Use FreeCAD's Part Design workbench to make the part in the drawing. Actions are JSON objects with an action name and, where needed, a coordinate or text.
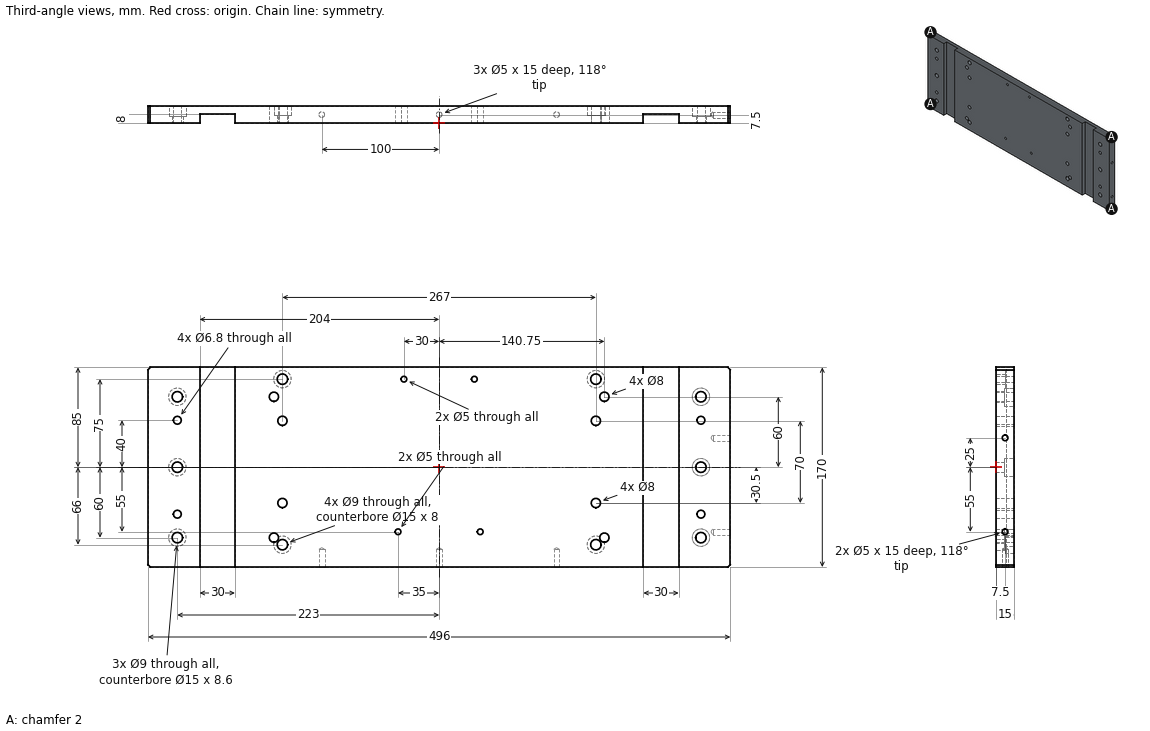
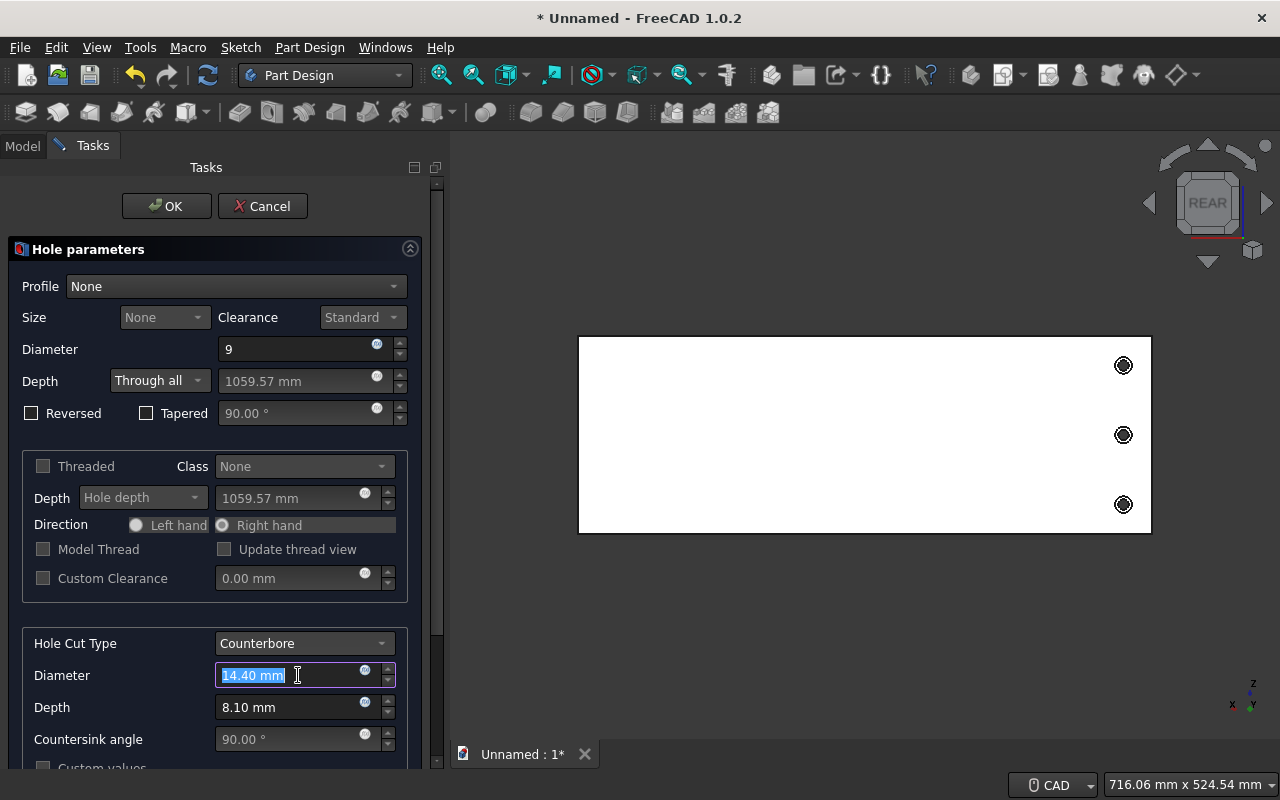
{"action": "type", "text": "15"}
{"action": "key", "text": "Tab"}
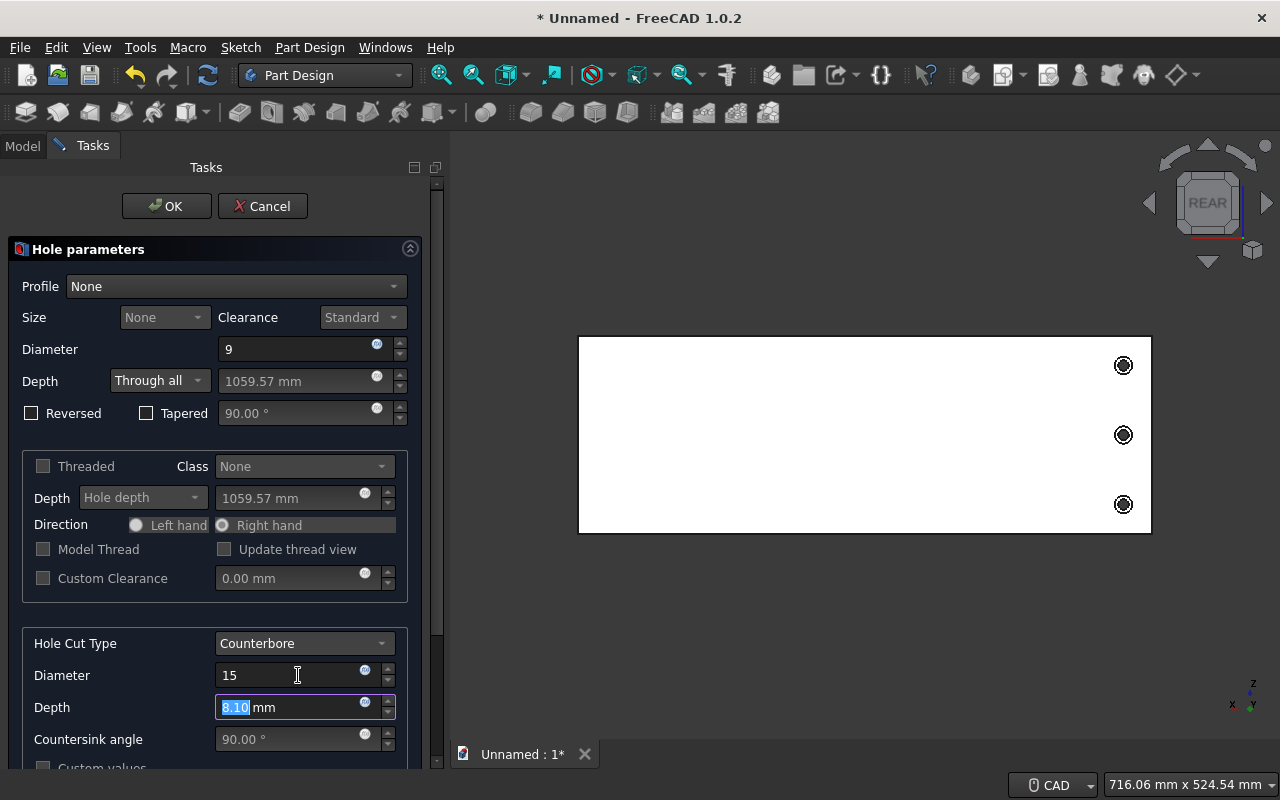
{"action": "type", "text": "8.6"}
{"action": "key", "text": "Tab"}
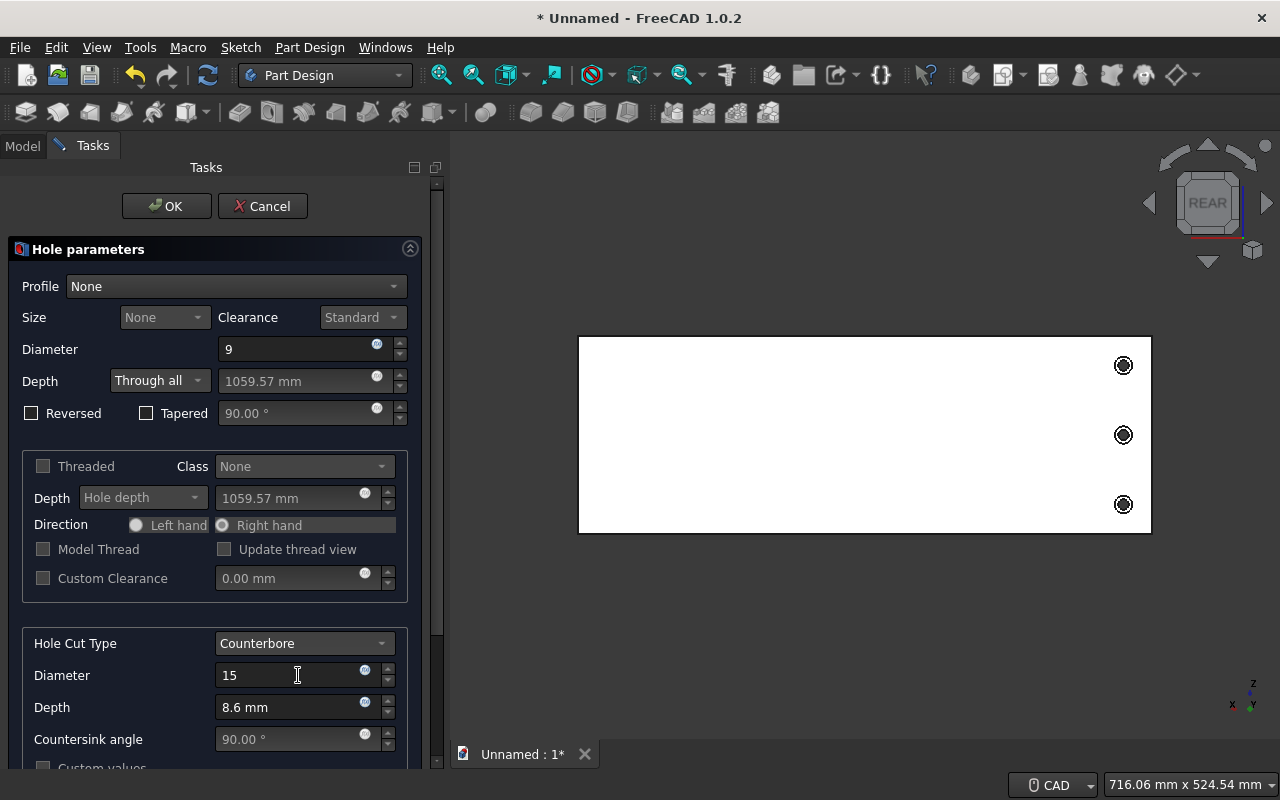
{"action": "left_click", "coordinate": [167, 206]}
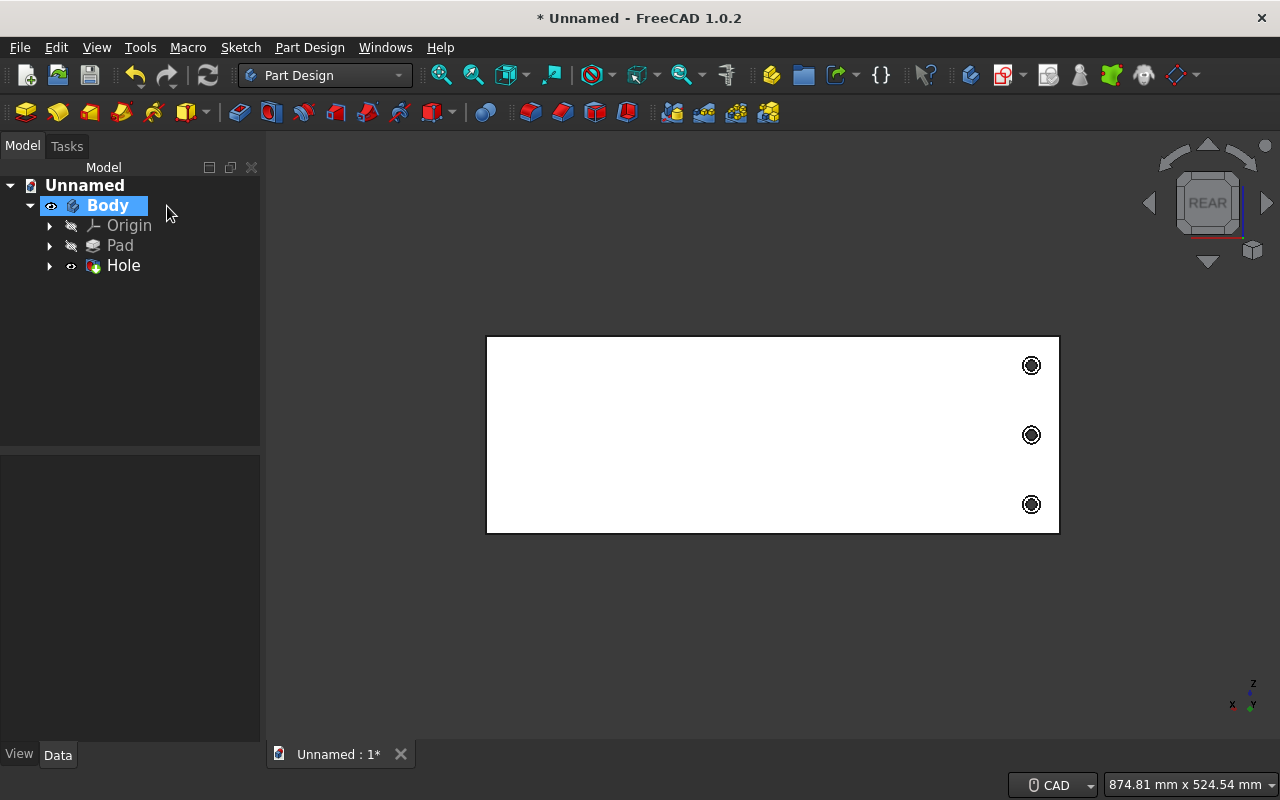
{"action": "key", "text": "0"}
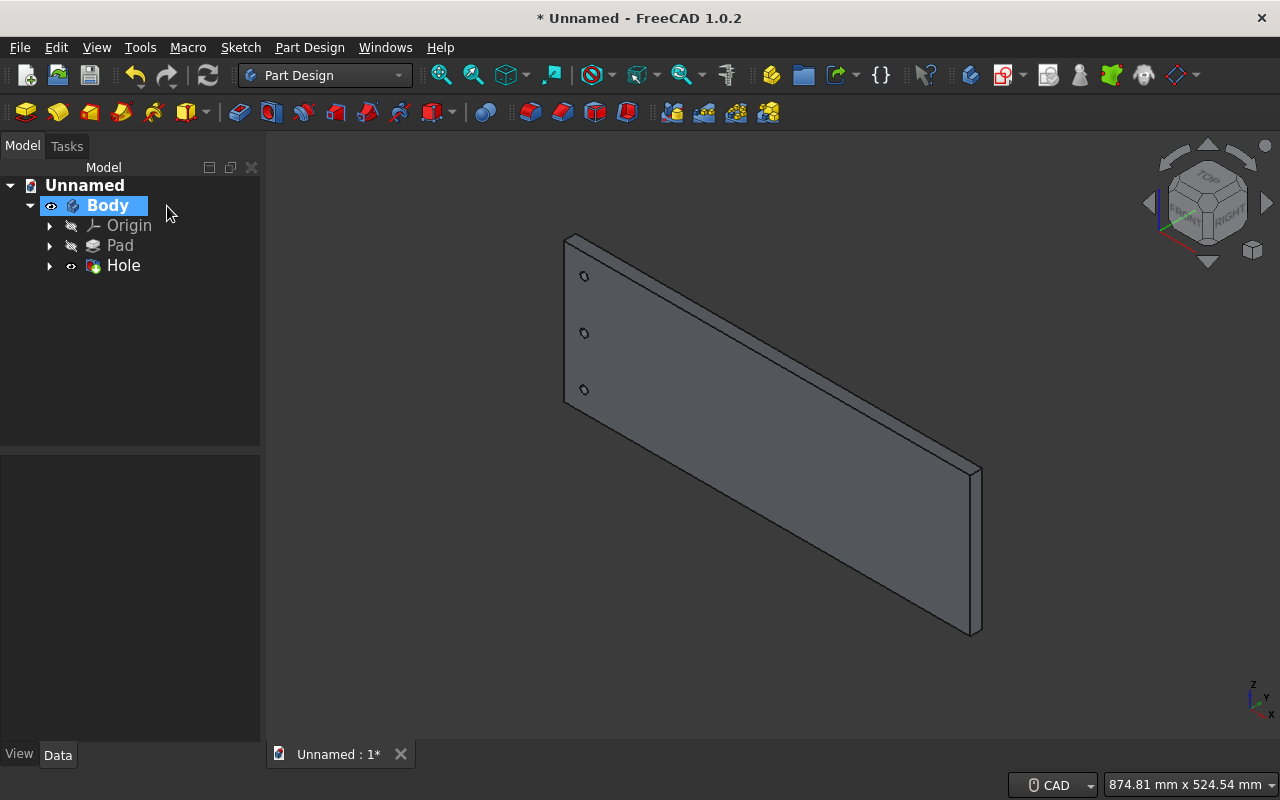
{"action": "left_click", "coordinate": [883, 505]}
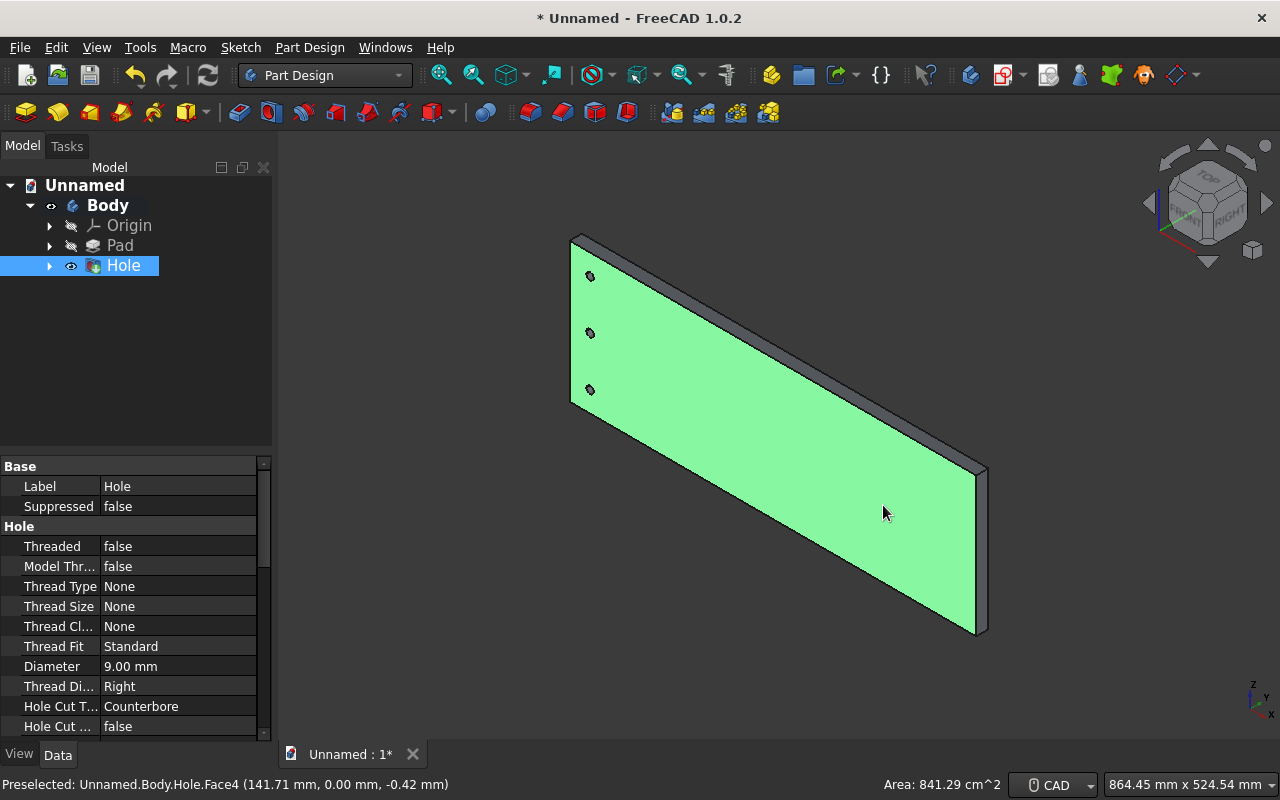
{"action": "left_click", "coordinate": [1004, 76]}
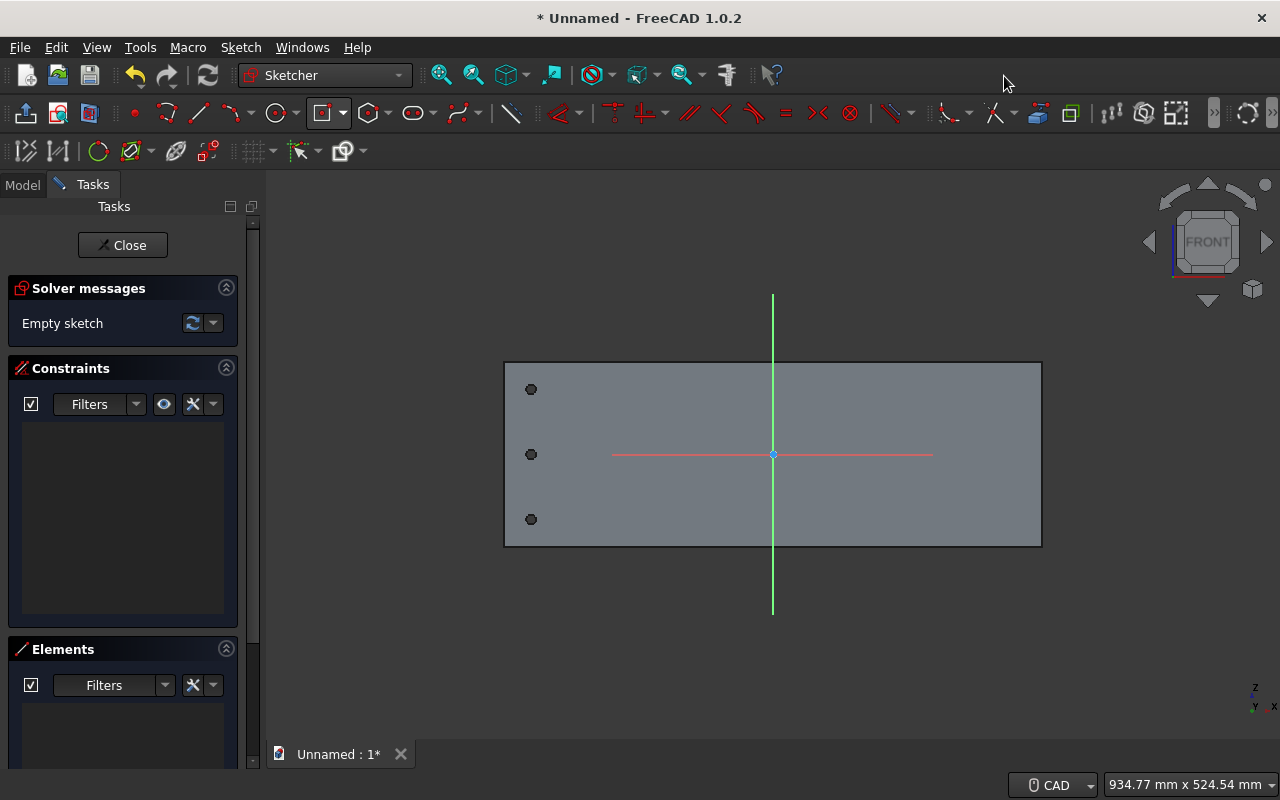
{"action": "scroll", "coordinate": [856, 455], "scroll_direction": "up", "scroll_amount": 3}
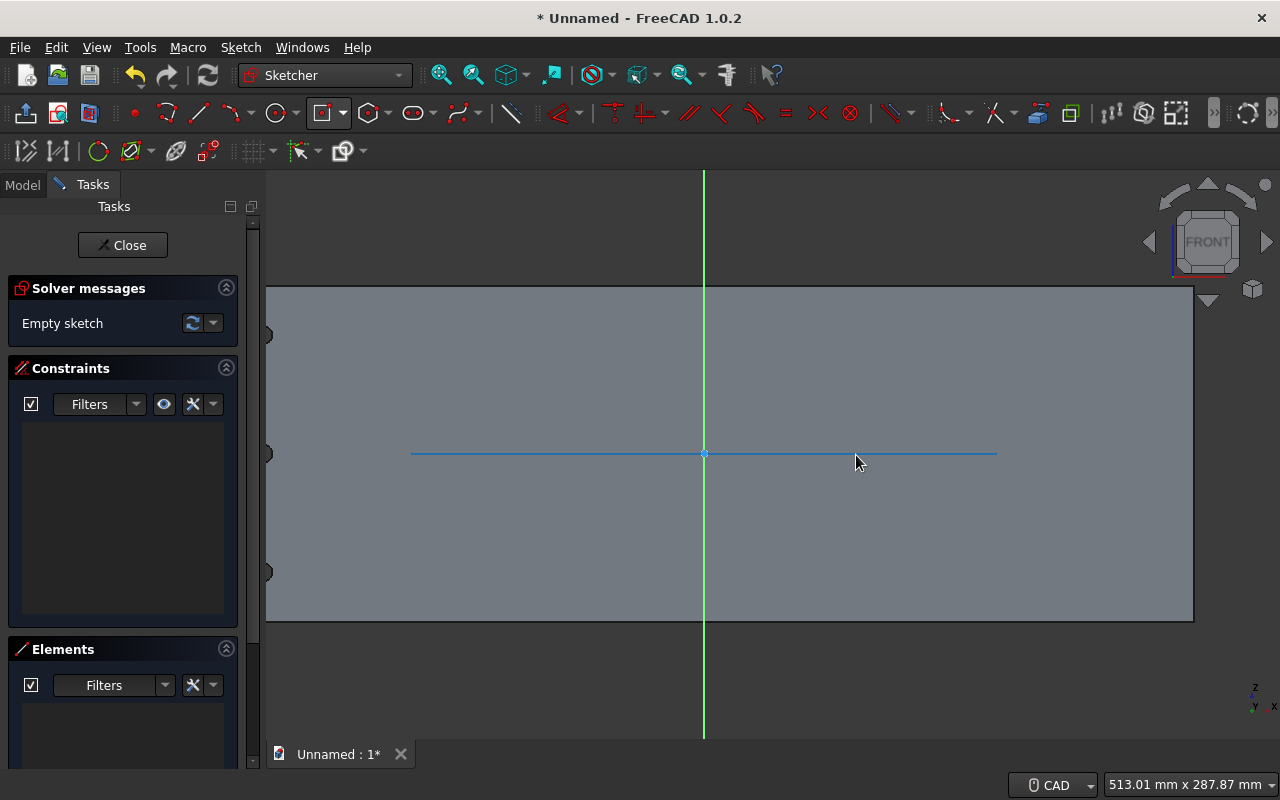
{"action": "left_click", "coordinate": [276, 114]}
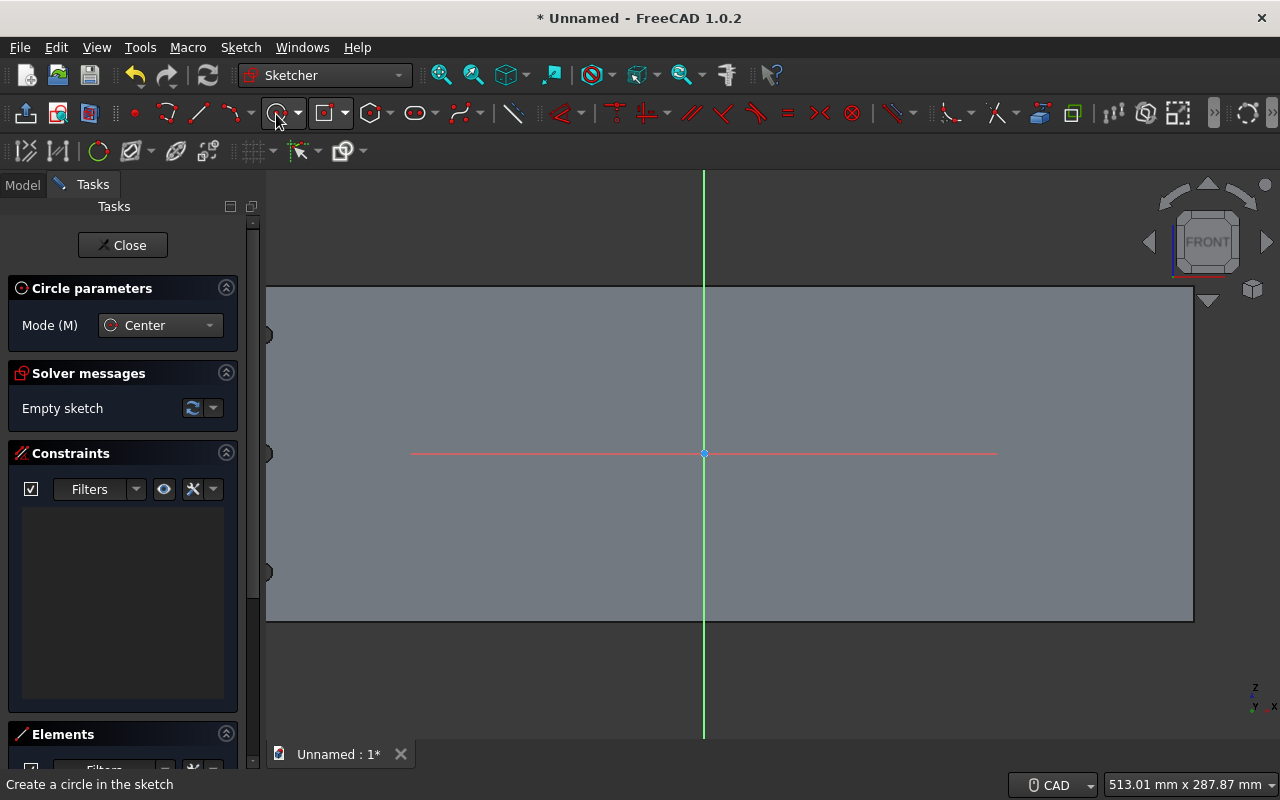
{"action": "scroll", "coordinate": [982, 335], "scroll_direction": "up", "scroll_amount": 6}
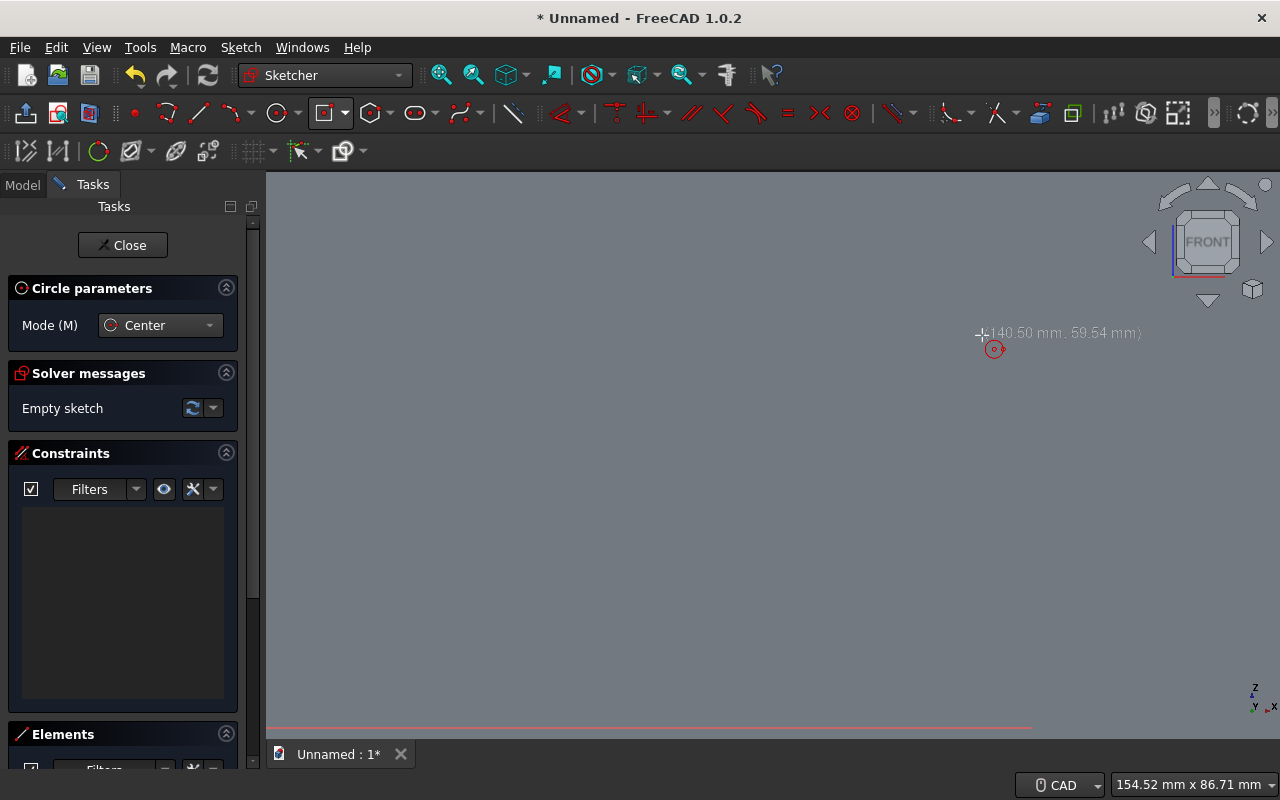
{"action": "left_click", "coordinate": [982, 335]}
{"action": "mouse_move", "coordinate": [1001, 316]}